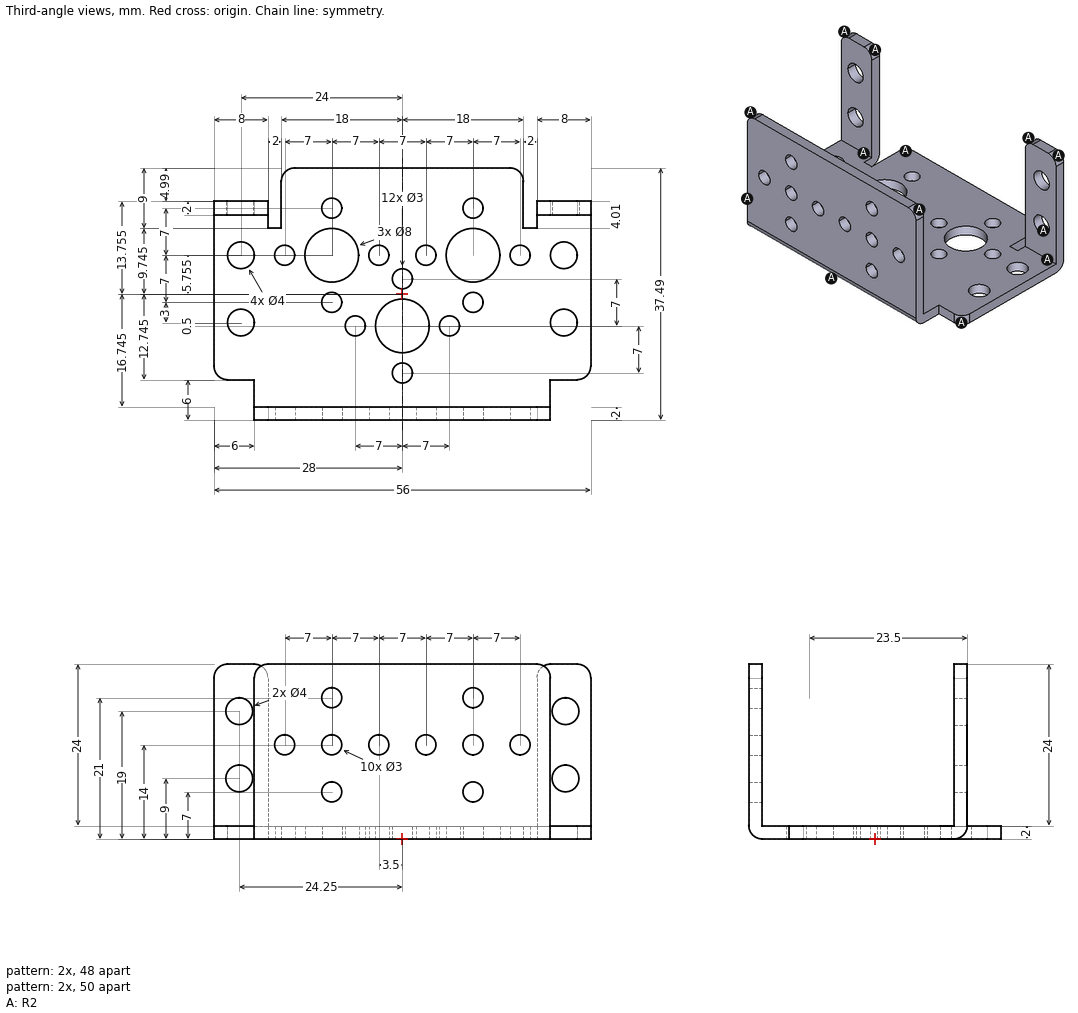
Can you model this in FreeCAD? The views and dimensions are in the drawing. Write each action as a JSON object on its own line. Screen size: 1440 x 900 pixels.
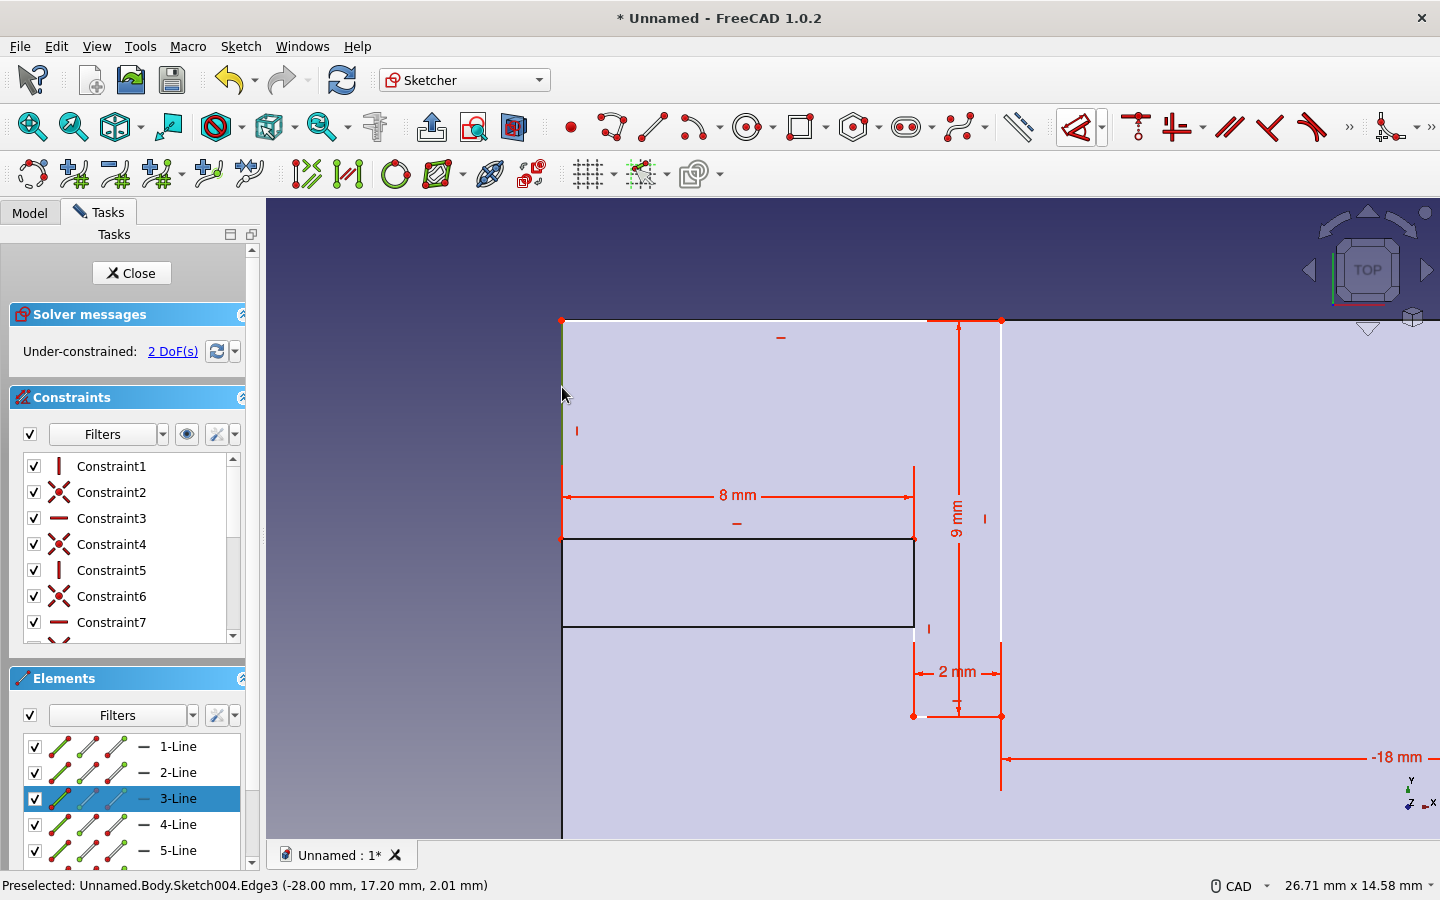
{"action": "key", "text": "i"}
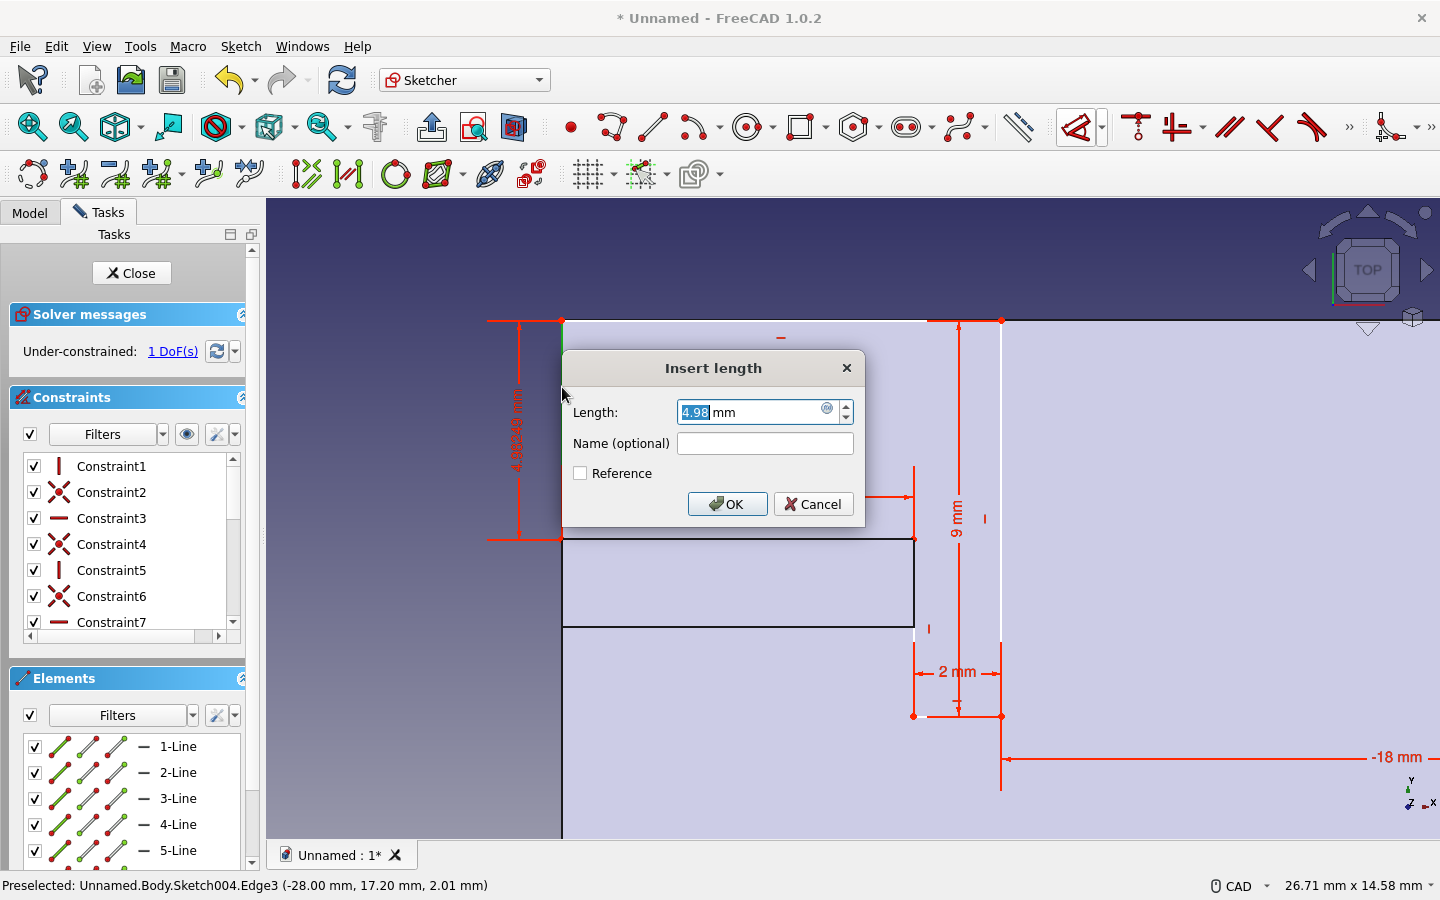
{"action": "type", "text": "4.99"}
{"action": "key", "text": "Return"}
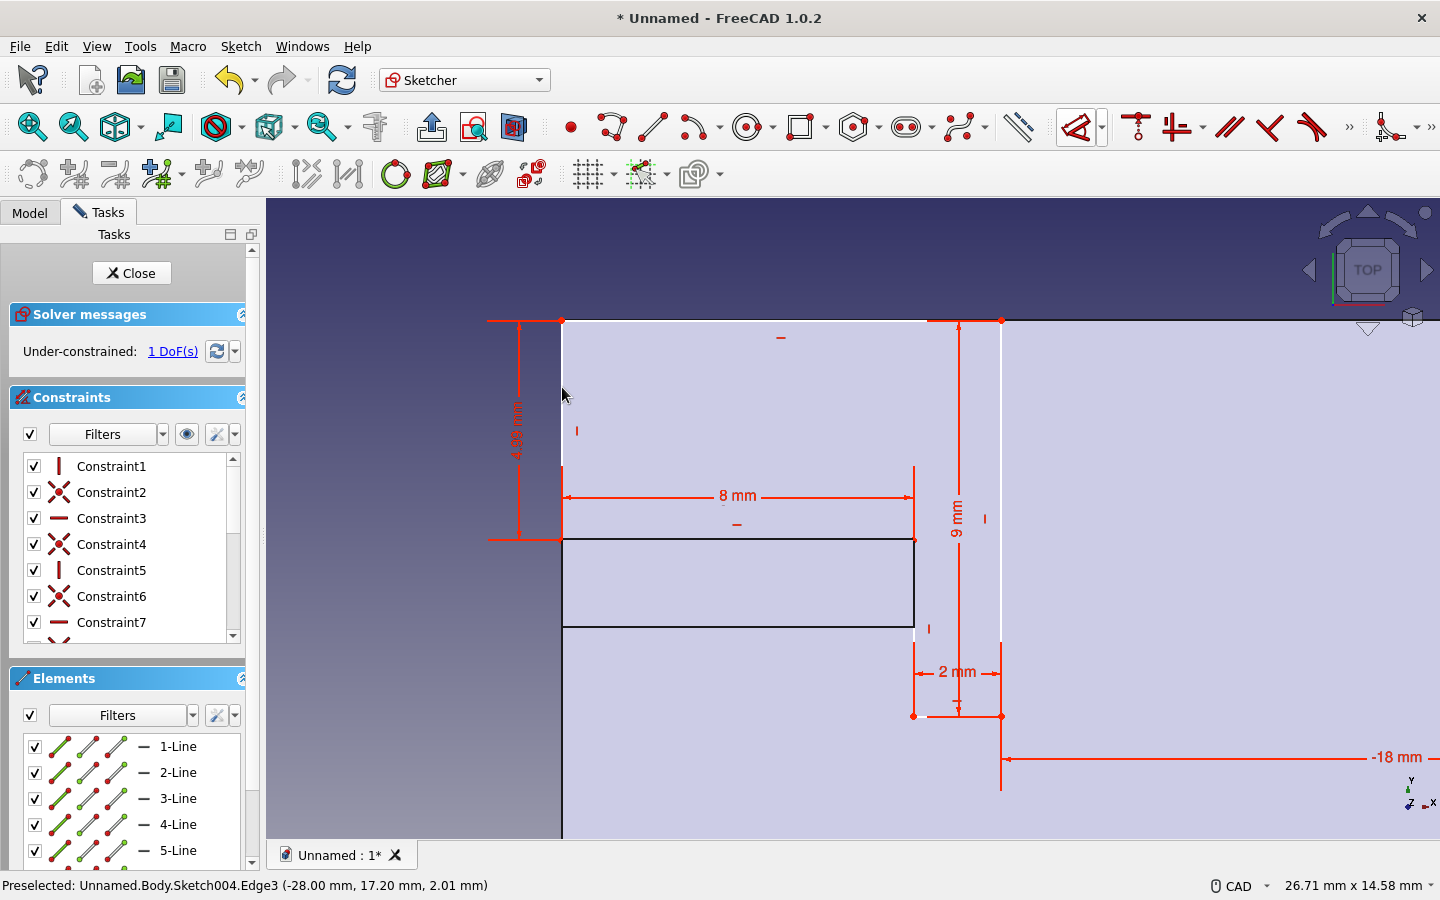
{"action": "left_click", "coordinate": [1001, 717]}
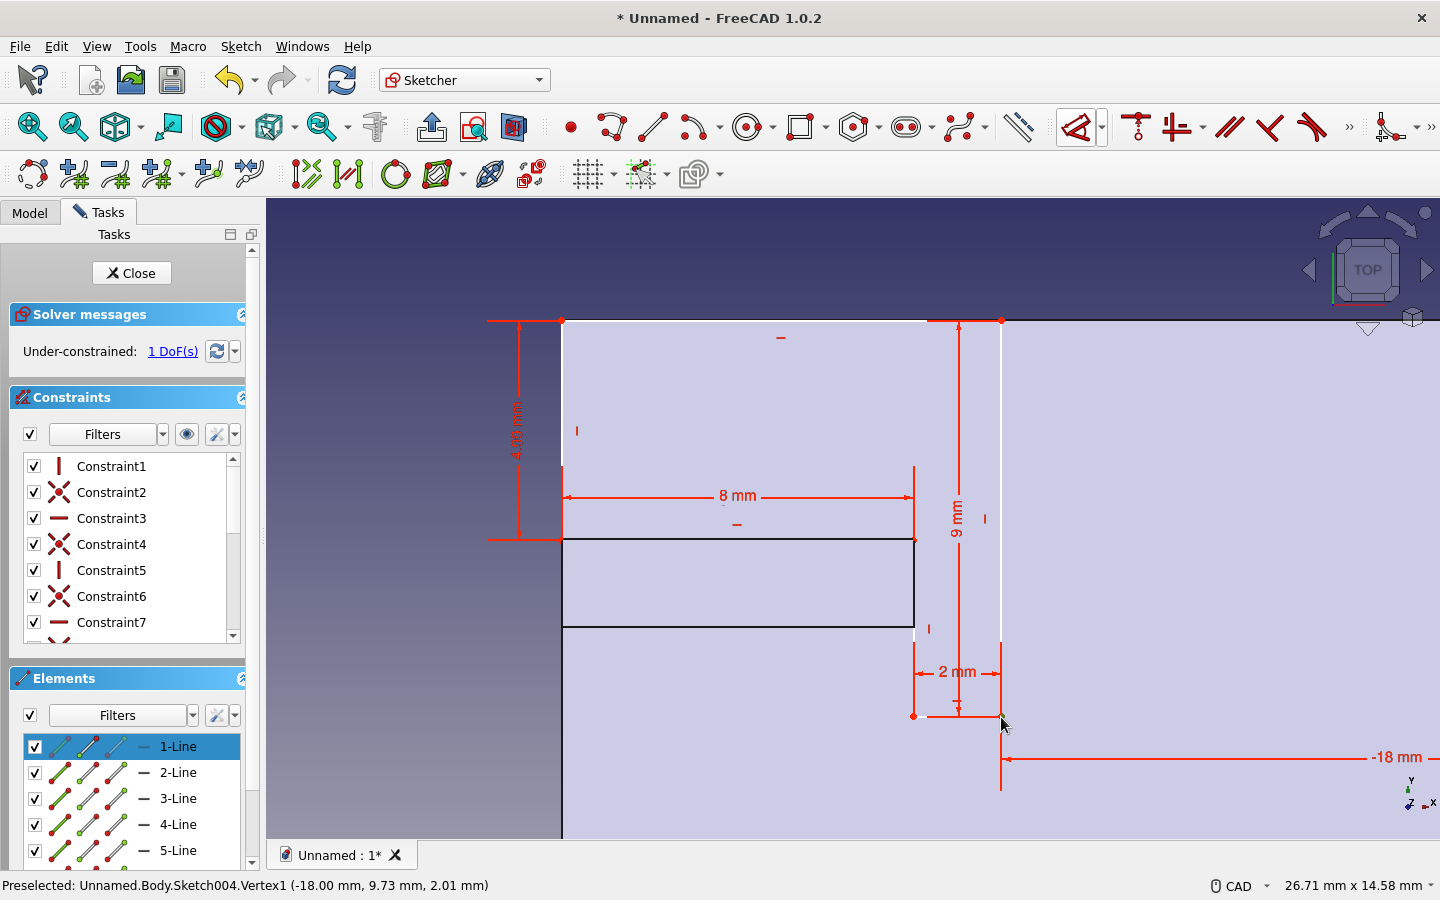
{"action": "key", "text": "i"}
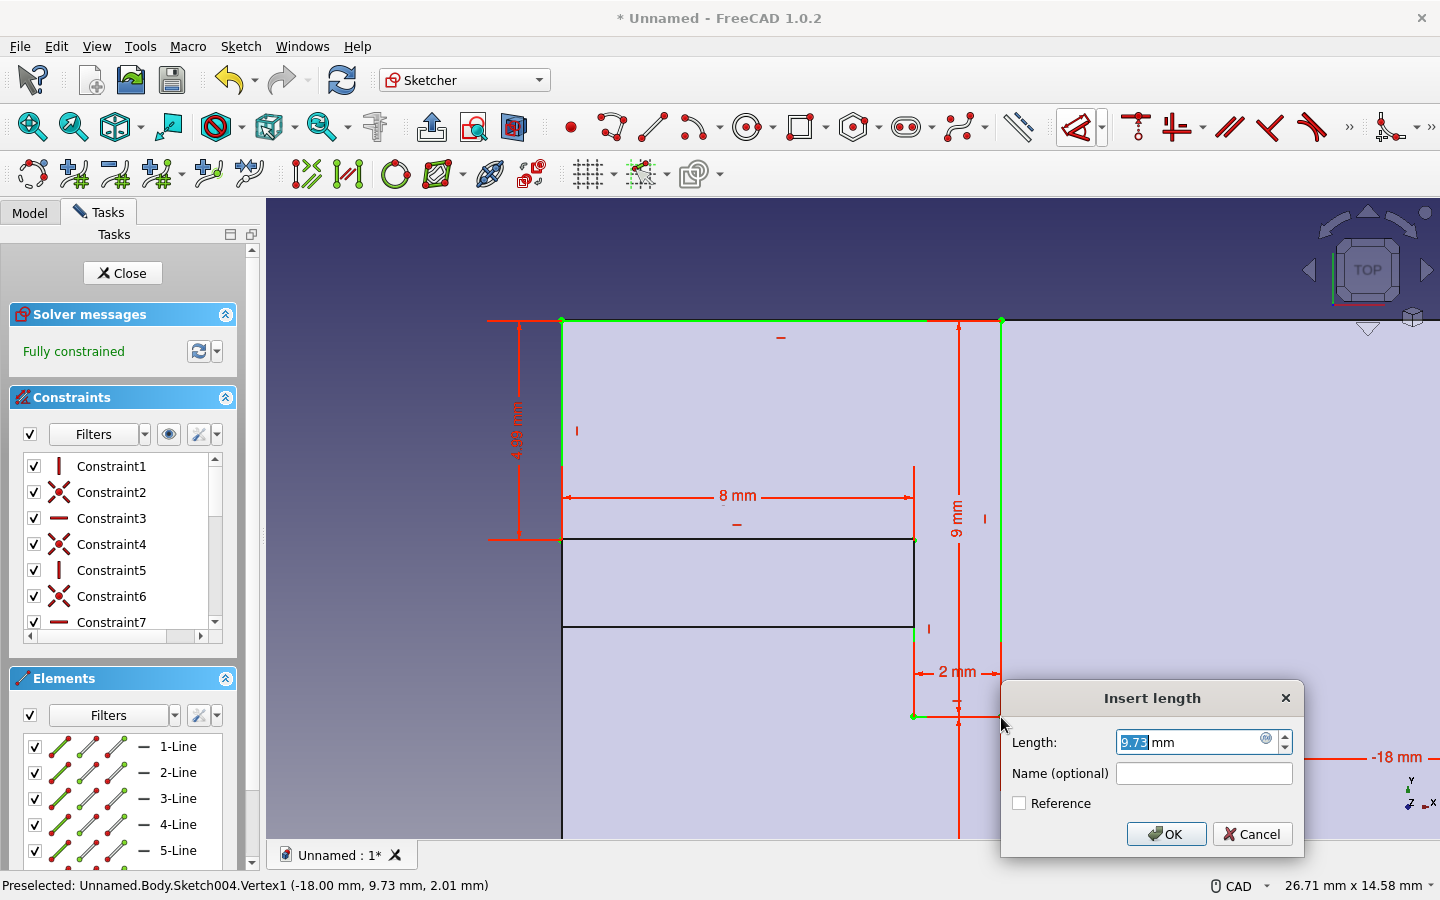
{"action": "type", "text": "9.745"}
{"action": "key", "text": "Return"}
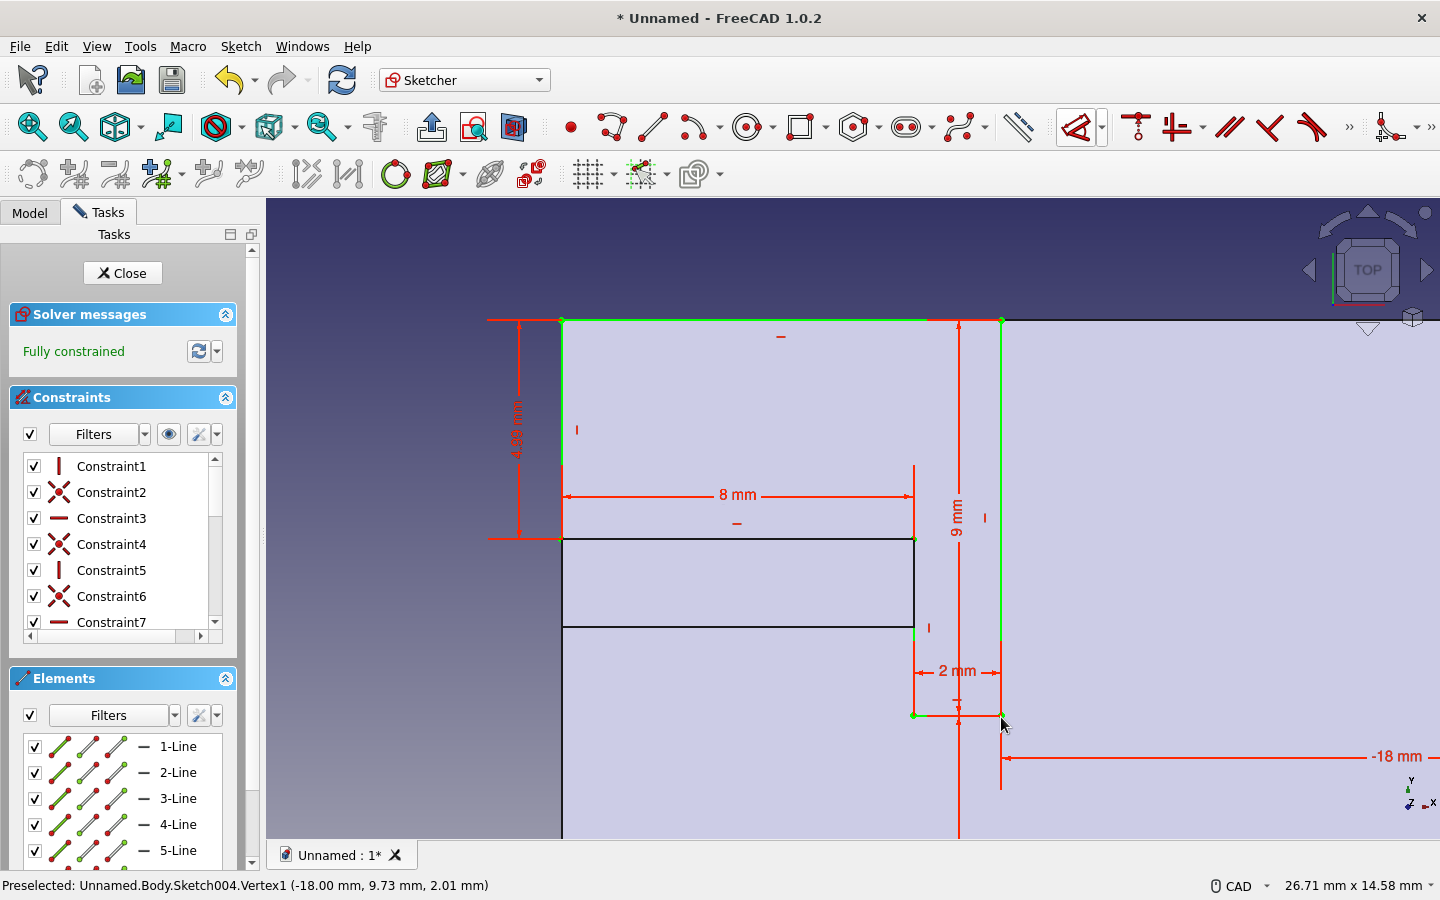
{"action": "left_click", "coordinate": [123, 273]}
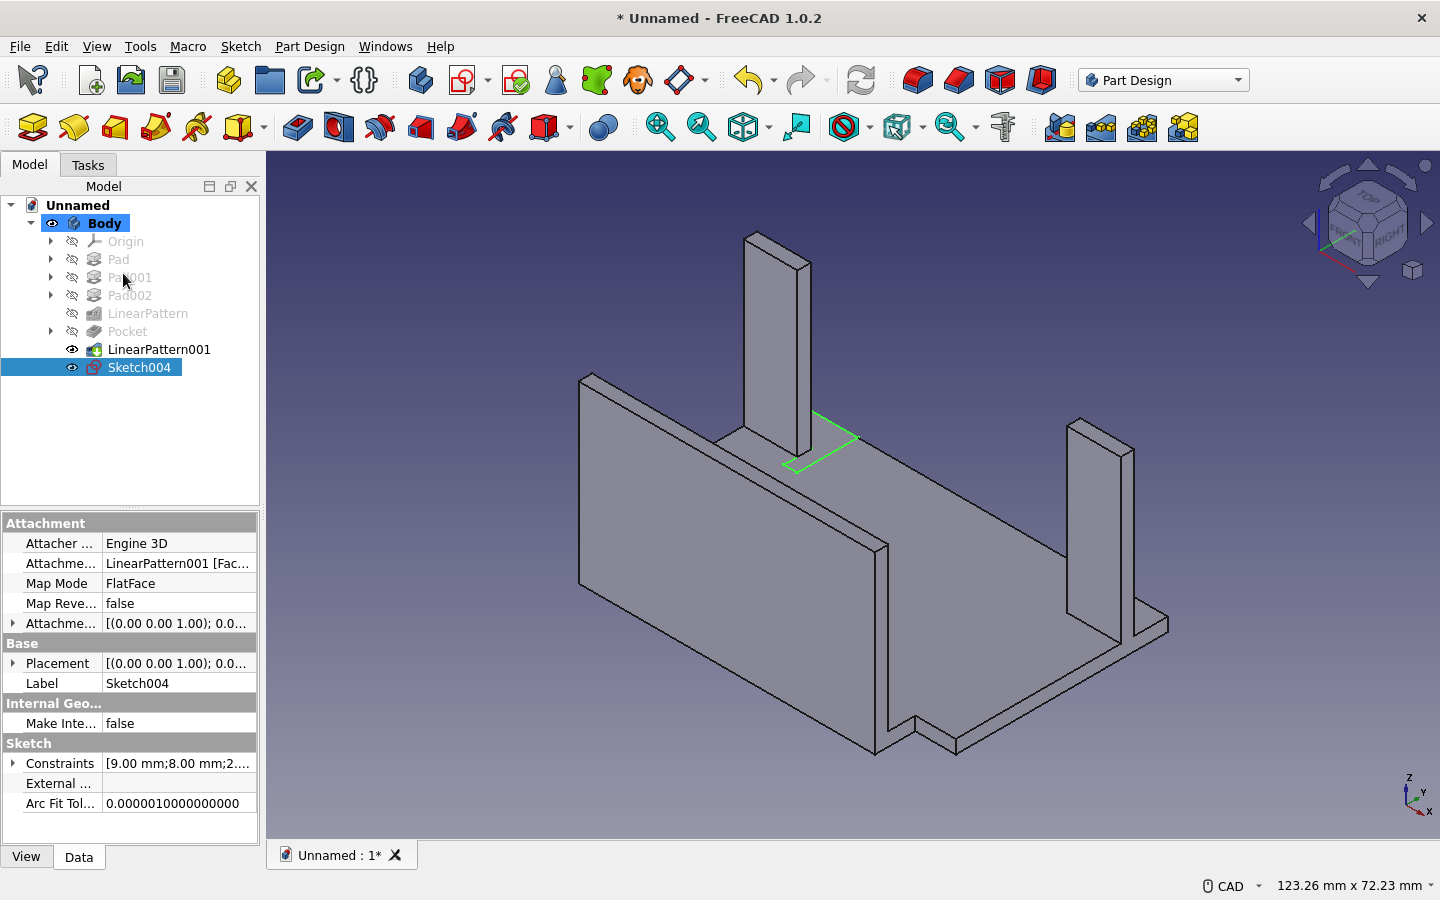
{"action": "left_click", "coordinate": [298, 128]}